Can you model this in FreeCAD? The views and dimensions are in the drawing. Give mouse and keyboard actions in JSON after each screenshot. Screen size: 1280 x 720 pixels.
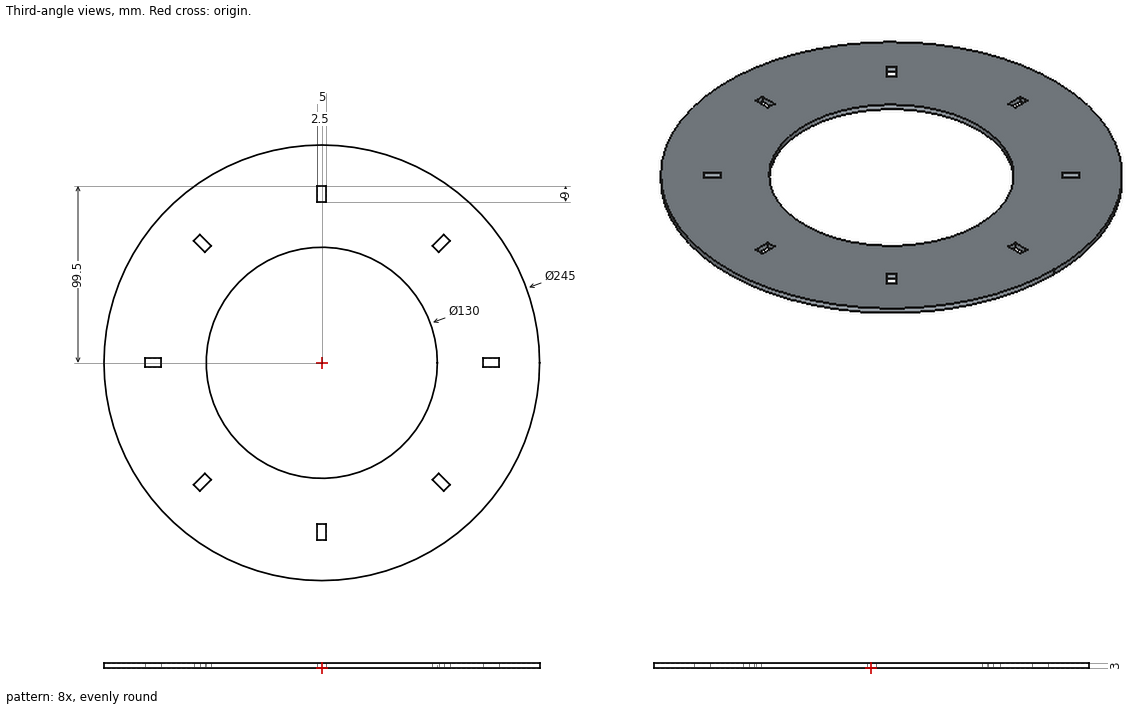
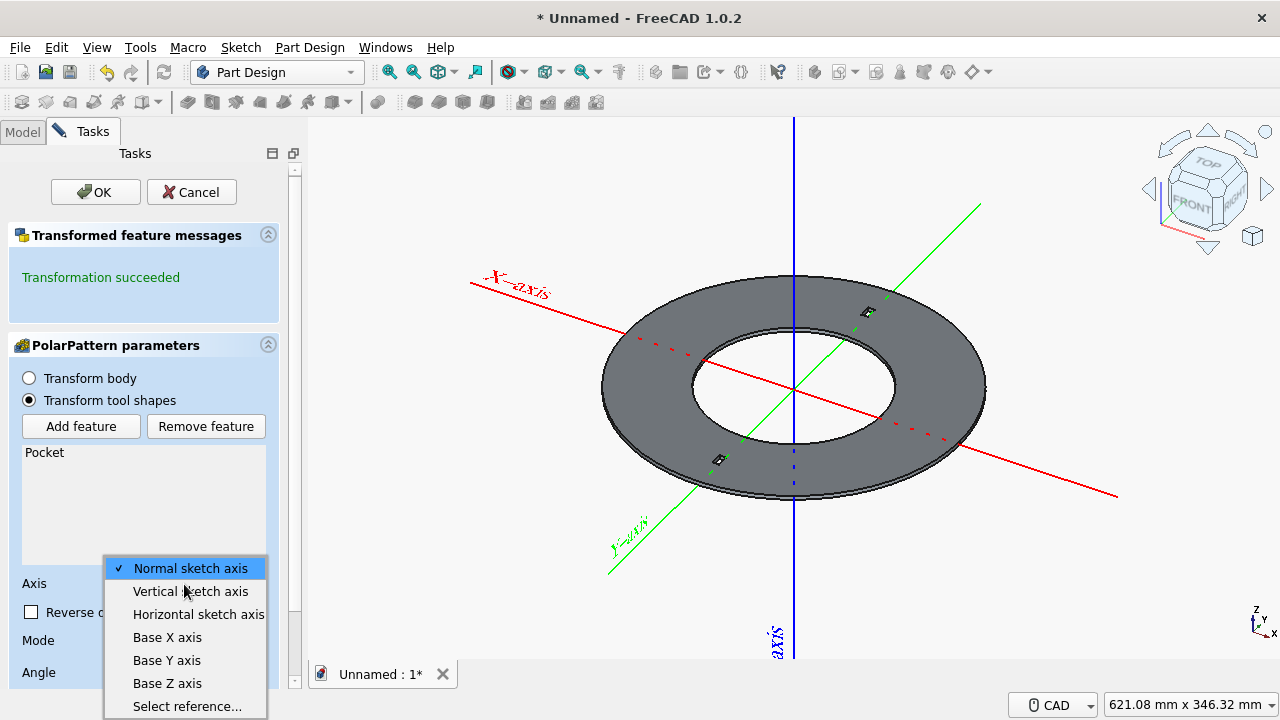
{"action": "left_click", "coordinate": [184, 684]}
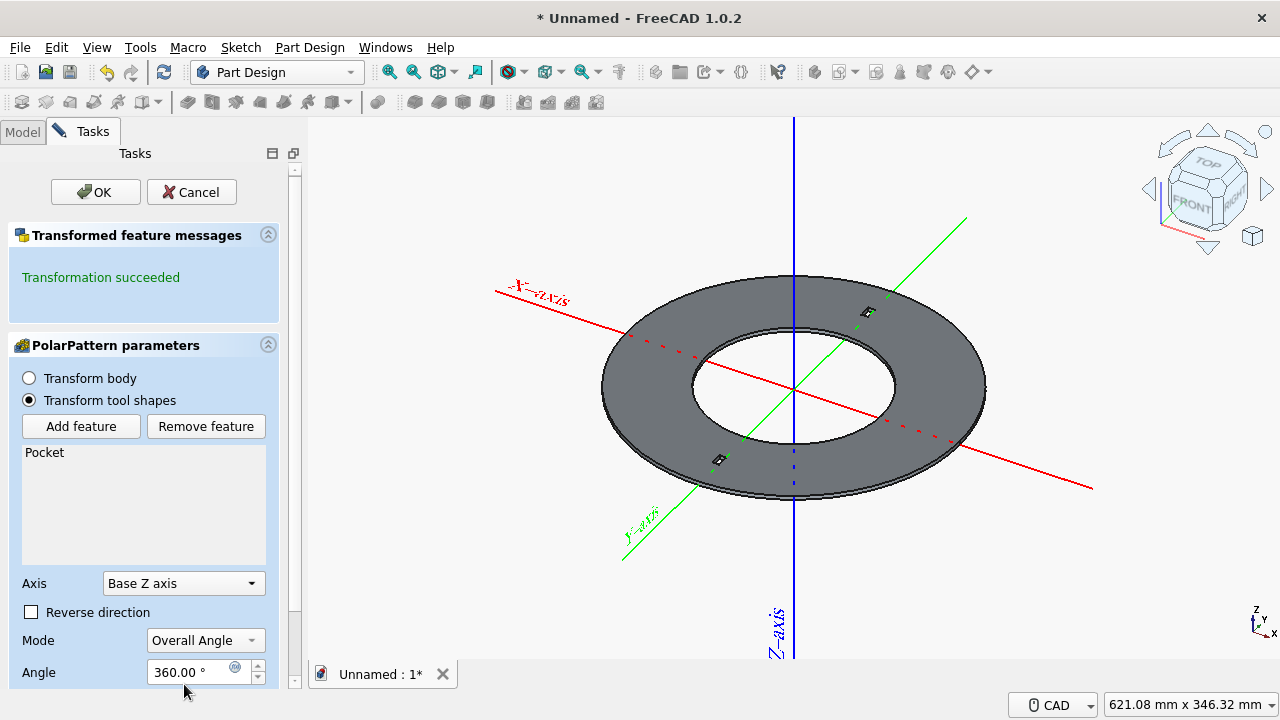
{"action": "scroll", "coordinate": [295, 426], "scroll_direction": "down", "scroll_amount": 2}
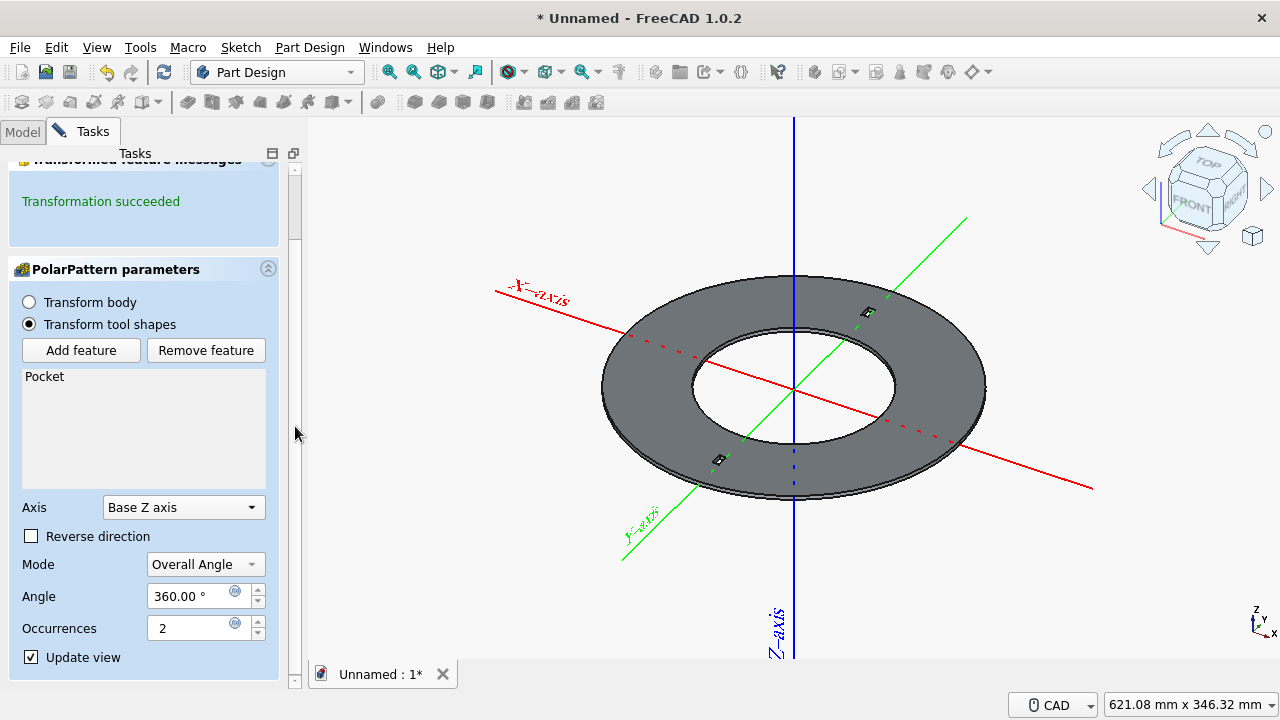
{"action": "triple_click", "coordinate": [198, 628]}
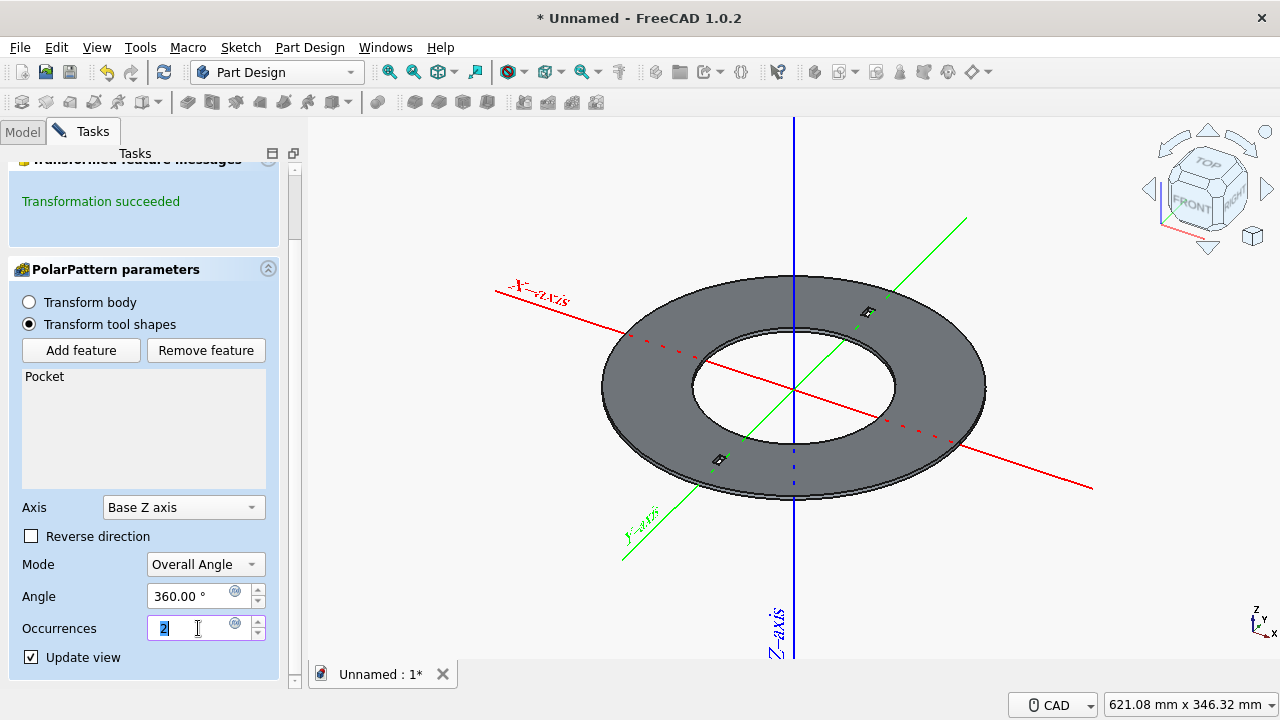
{"action": "type", "text": "8"}
{"action": "key", "text": "Tab"}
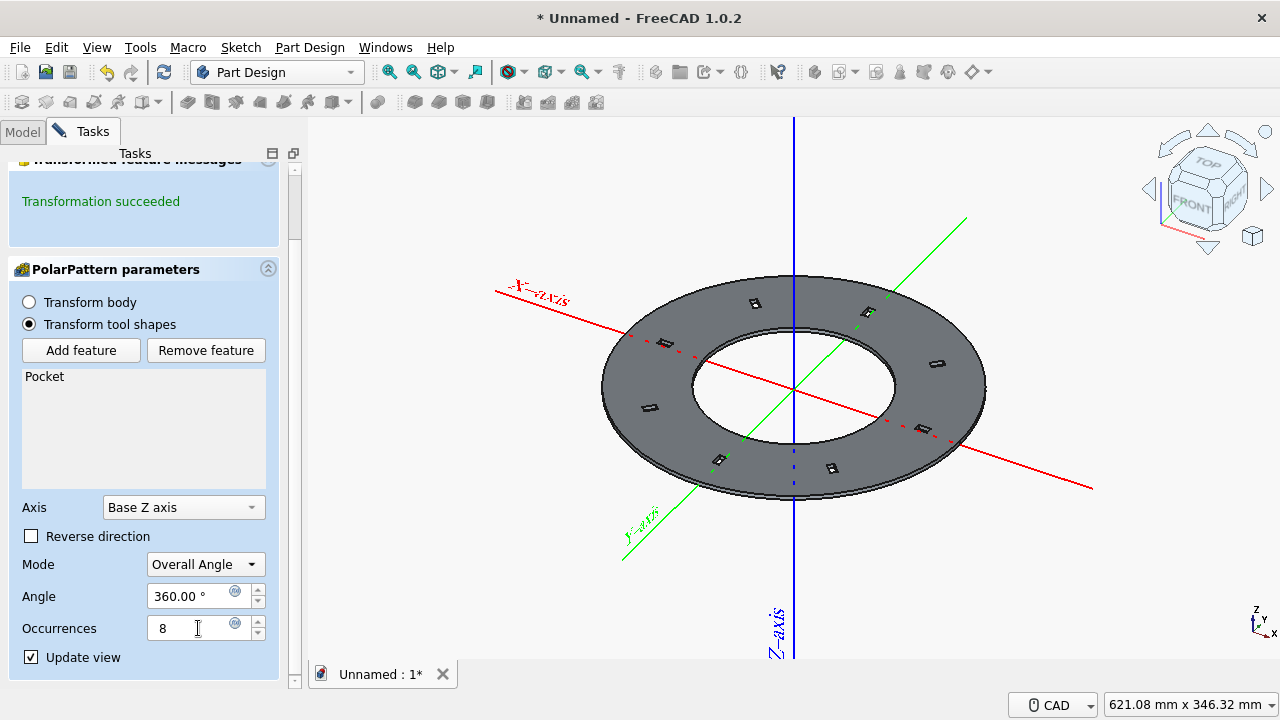
{"action": "scroll", "coordinate": [295, 426], "scroll_direction": "up", "scroll_amount": 3}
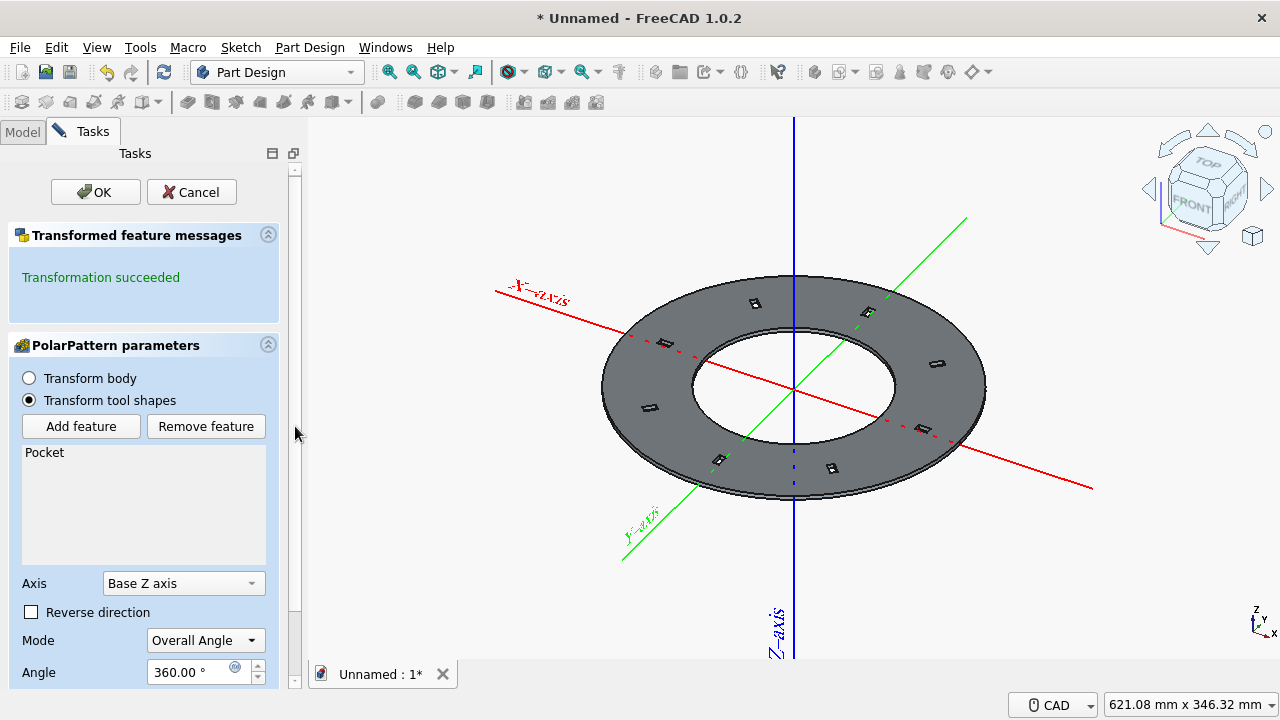
{"action": "left_click", "coordinate": [96, 192]}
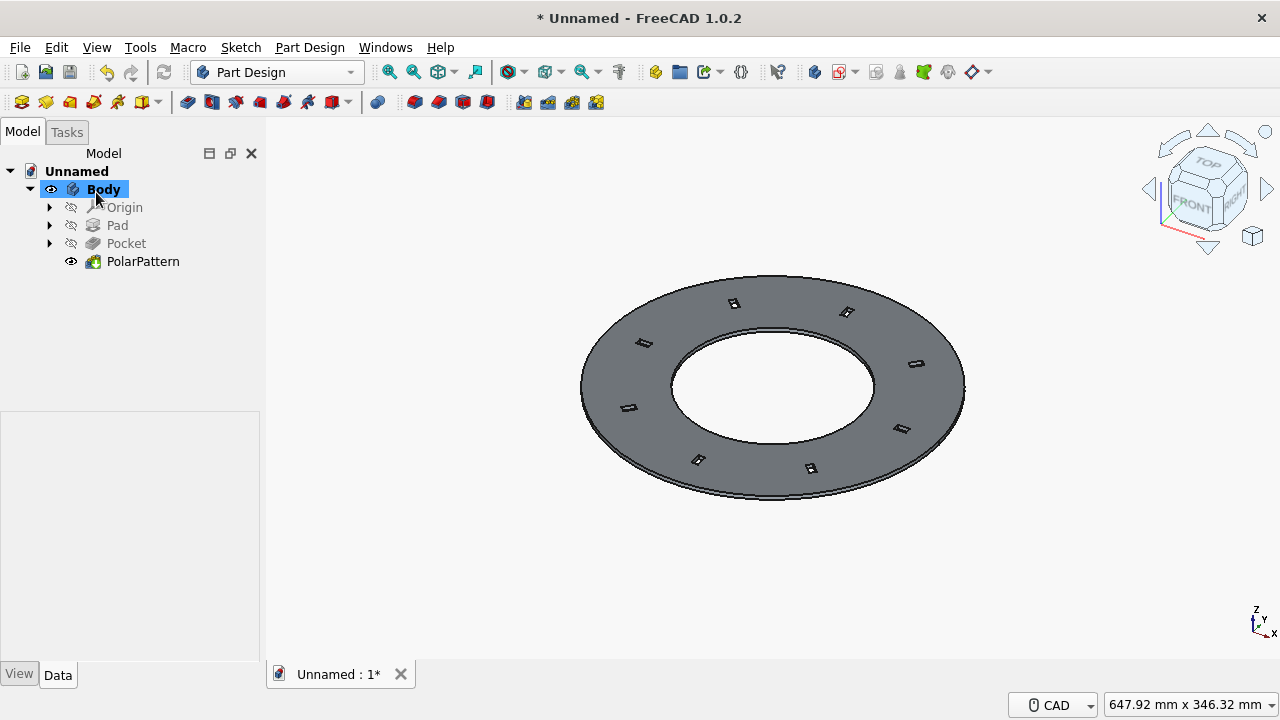
{"action": "key", "text": "0"}